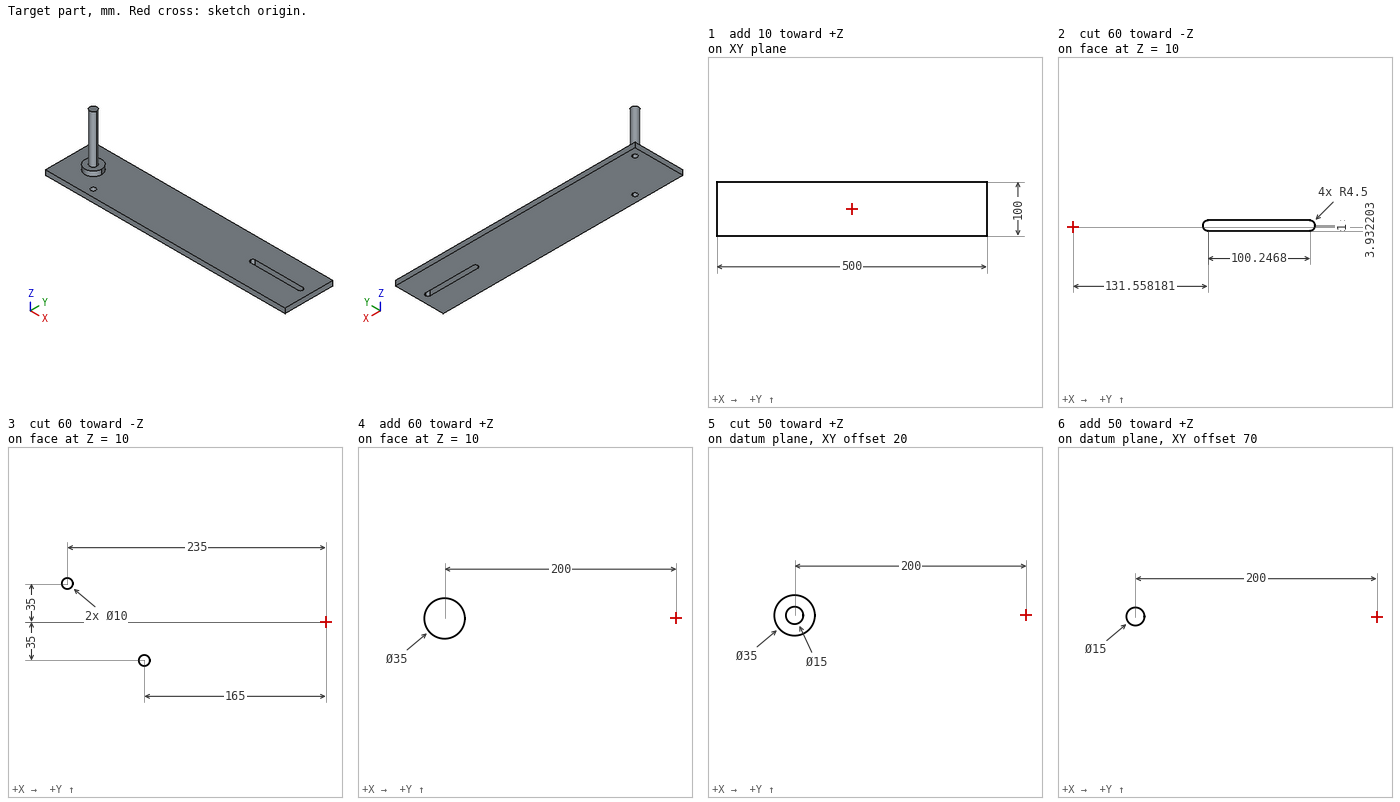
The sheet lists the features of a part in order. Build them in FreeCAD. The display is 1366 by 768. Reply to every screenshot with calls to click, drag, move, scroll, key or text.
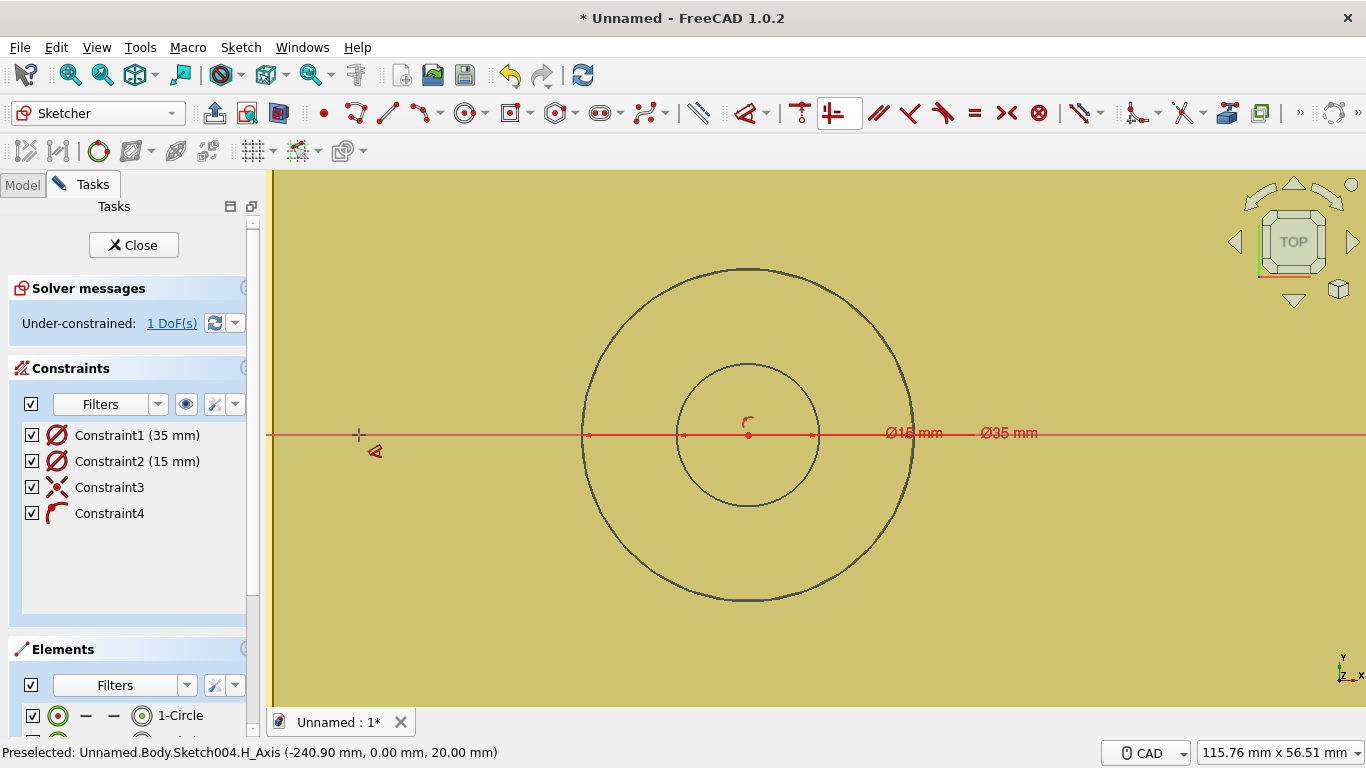
click(748, 435)
click(975, 469)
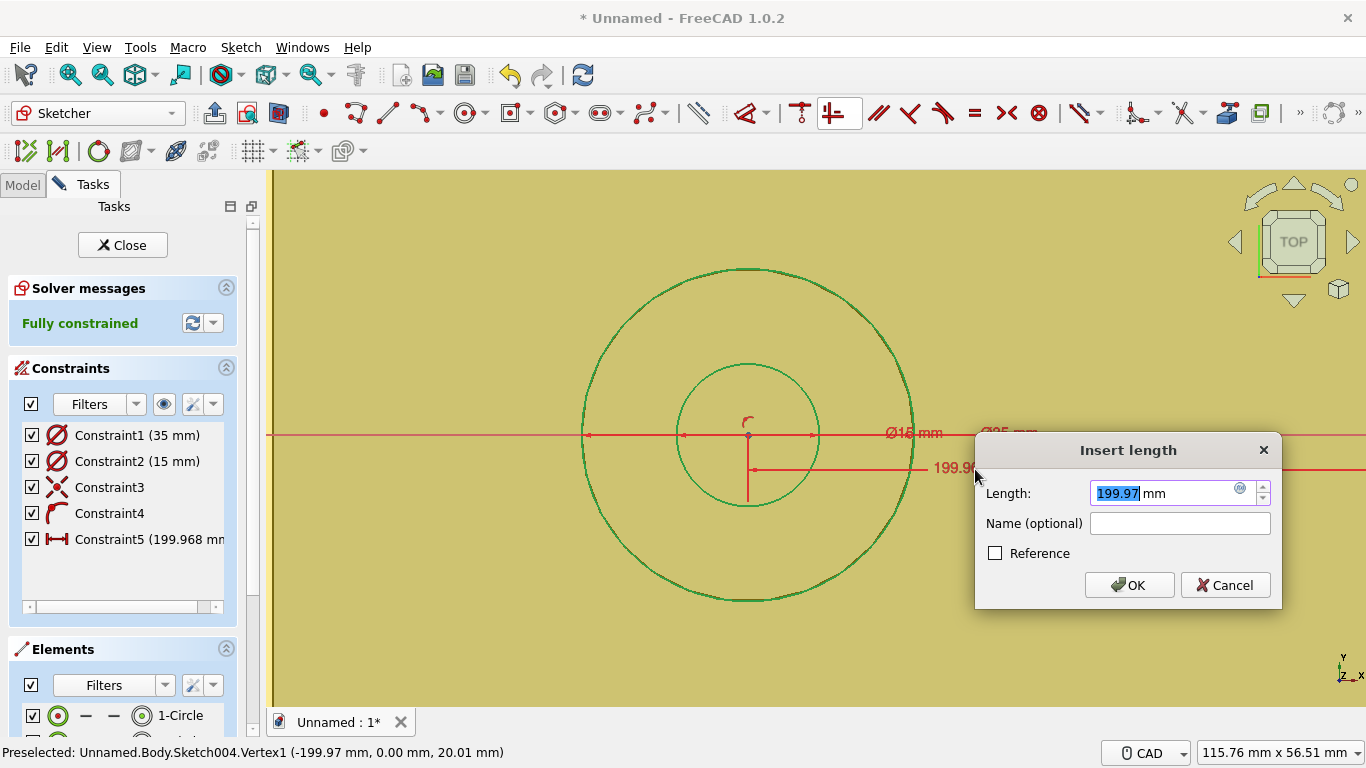
text(200)
key(Return)
key(Escape)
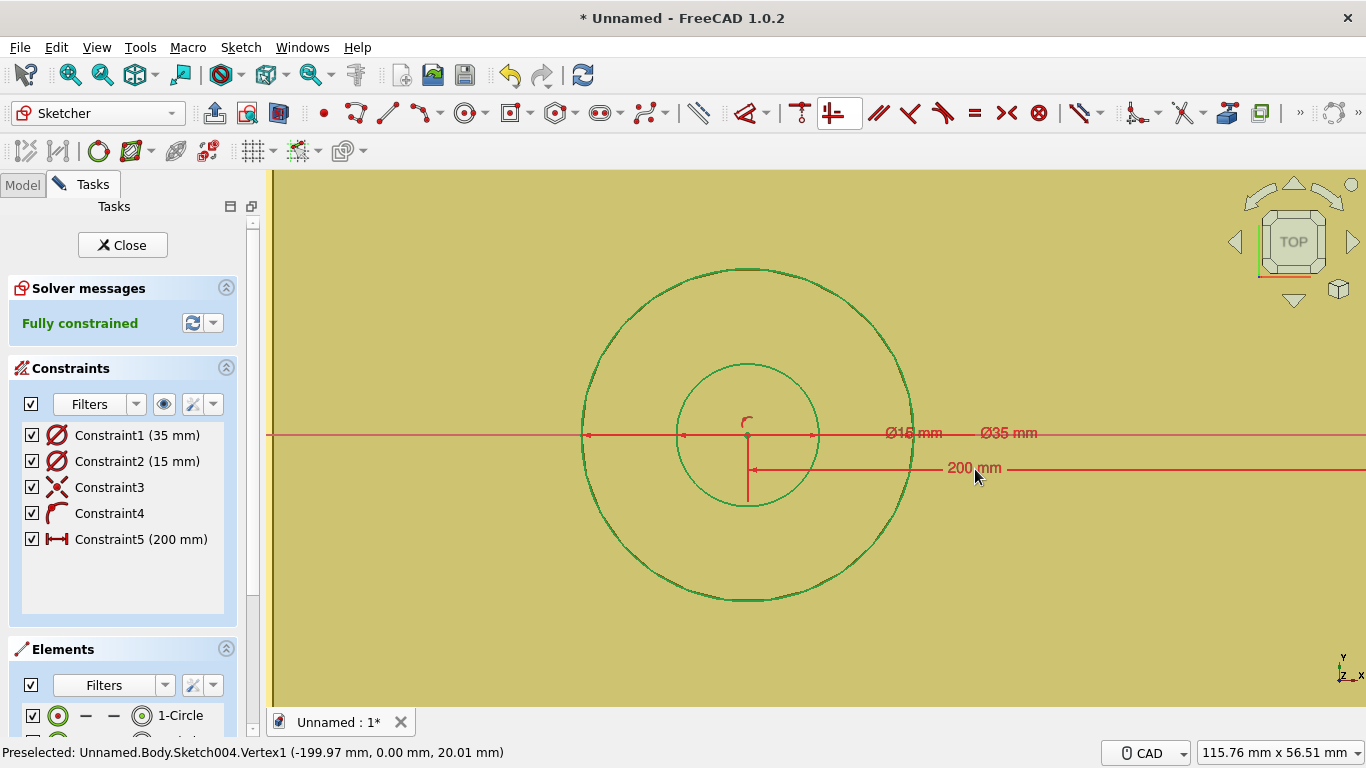
click(123, 245)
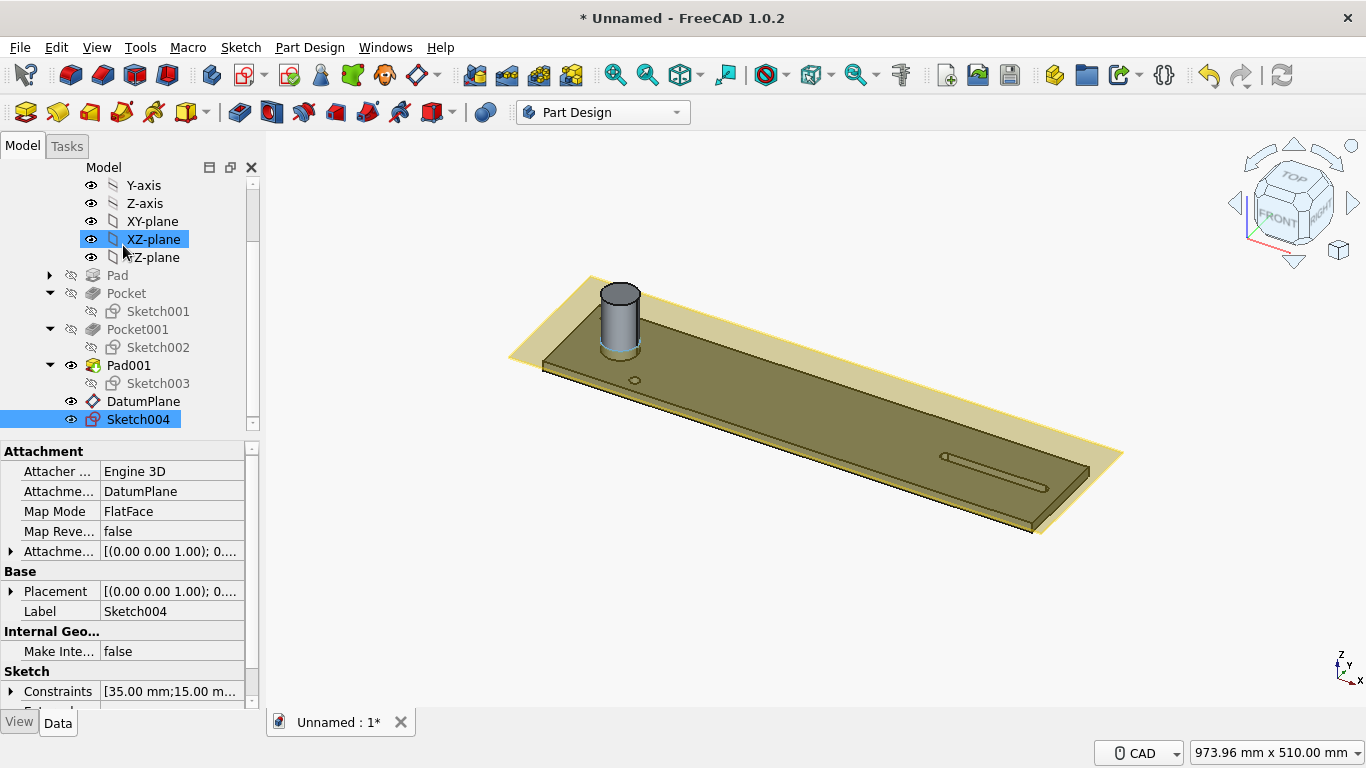
click(240, 112)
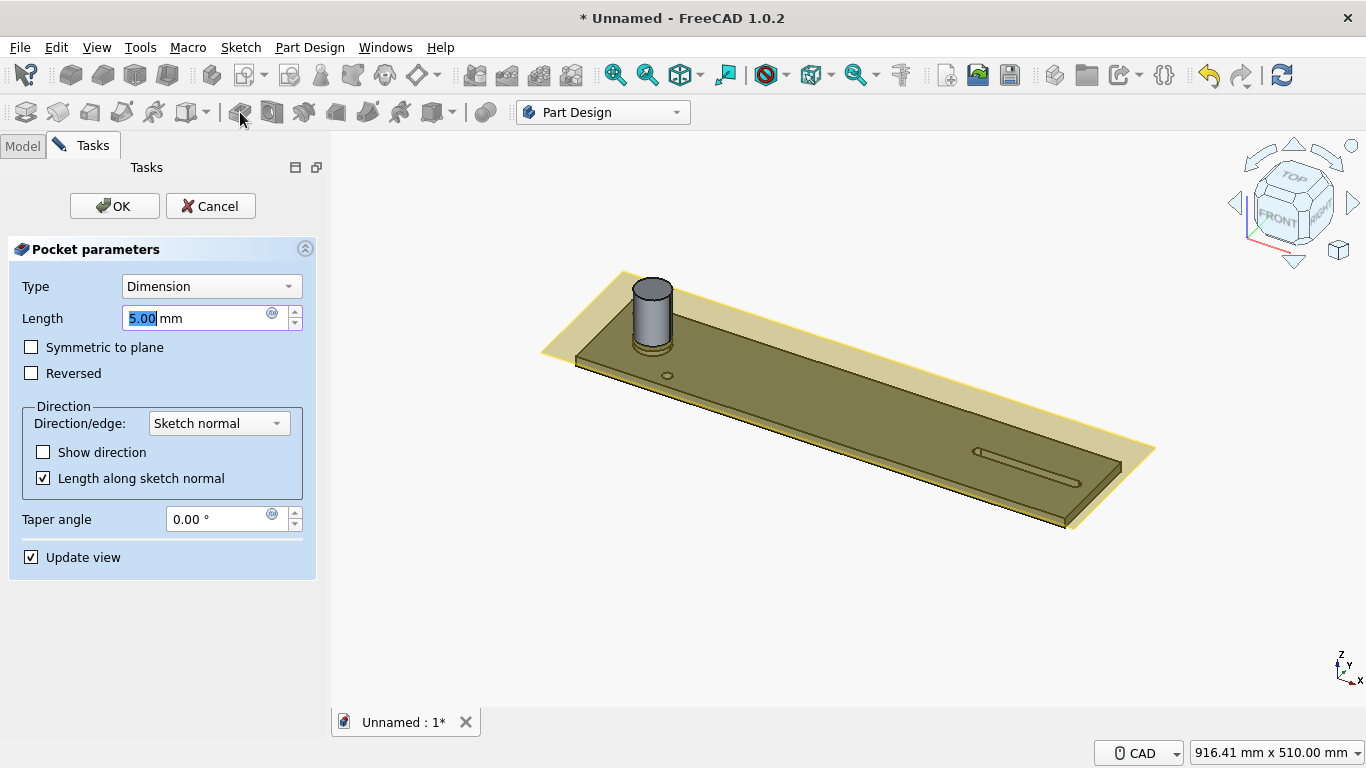
text(50)
key(Tab)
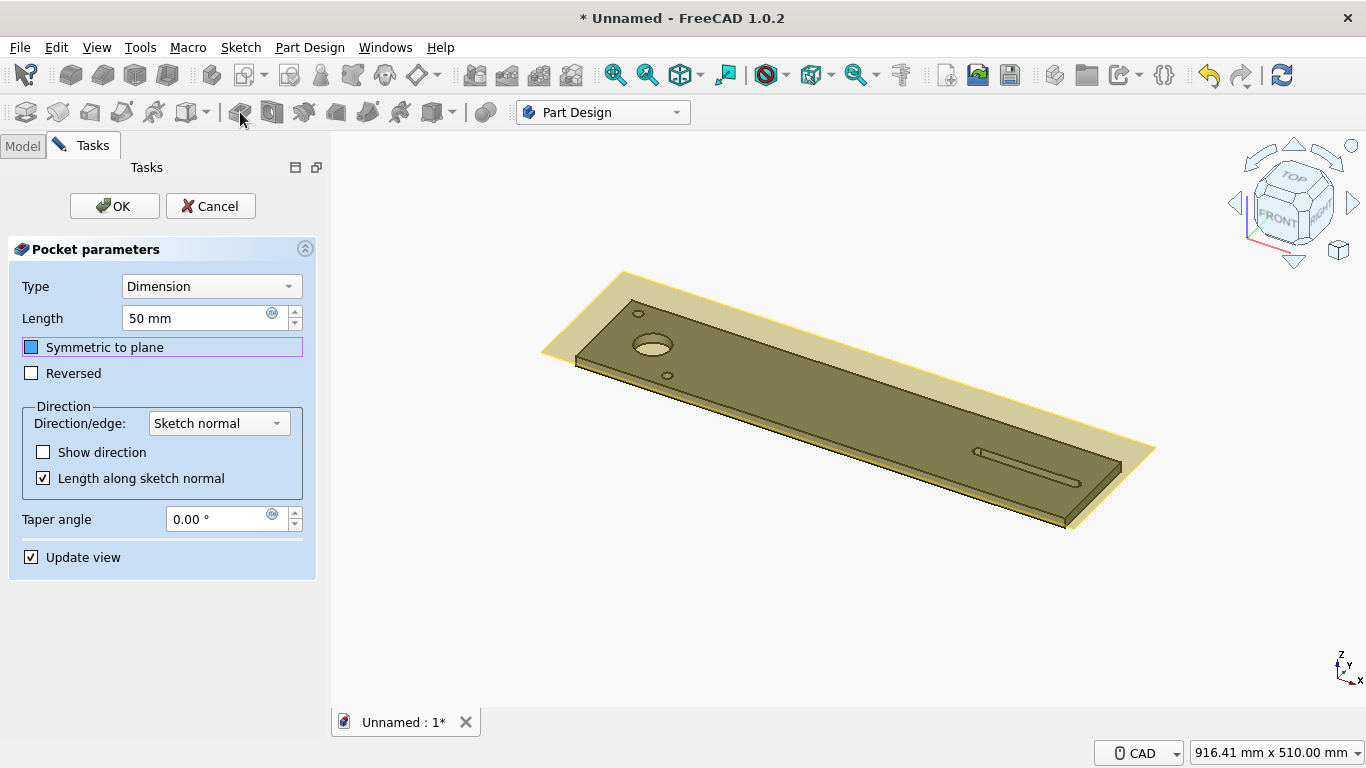
click(30, 373)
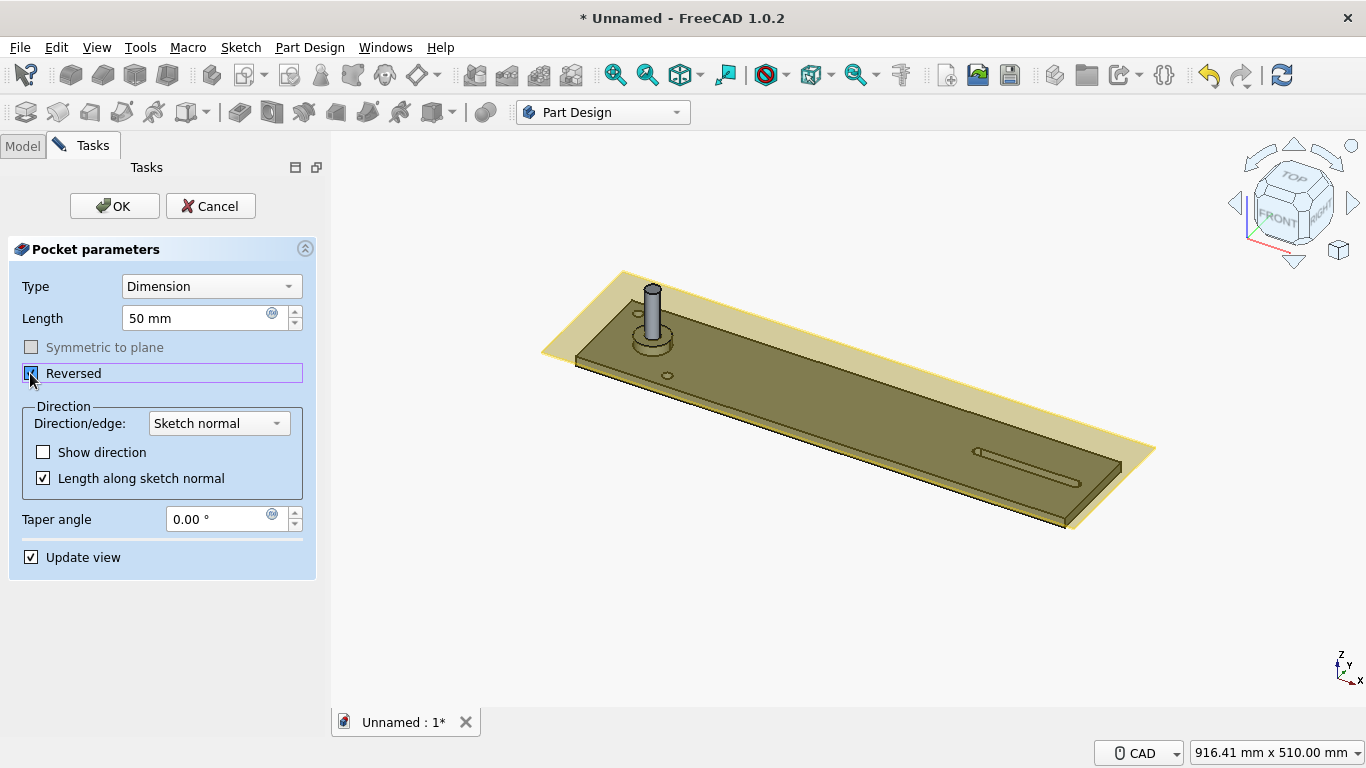
click(115, 206)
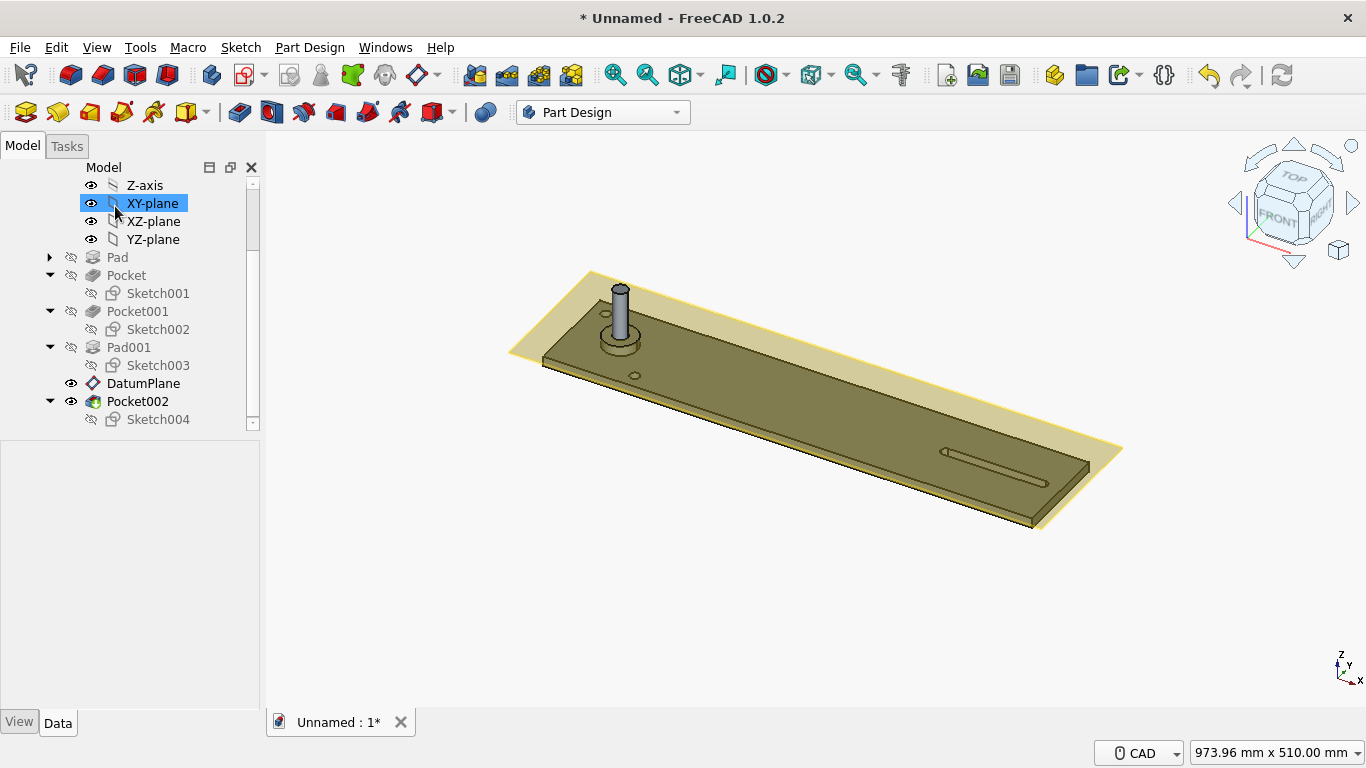
click(116, 383)
key(space)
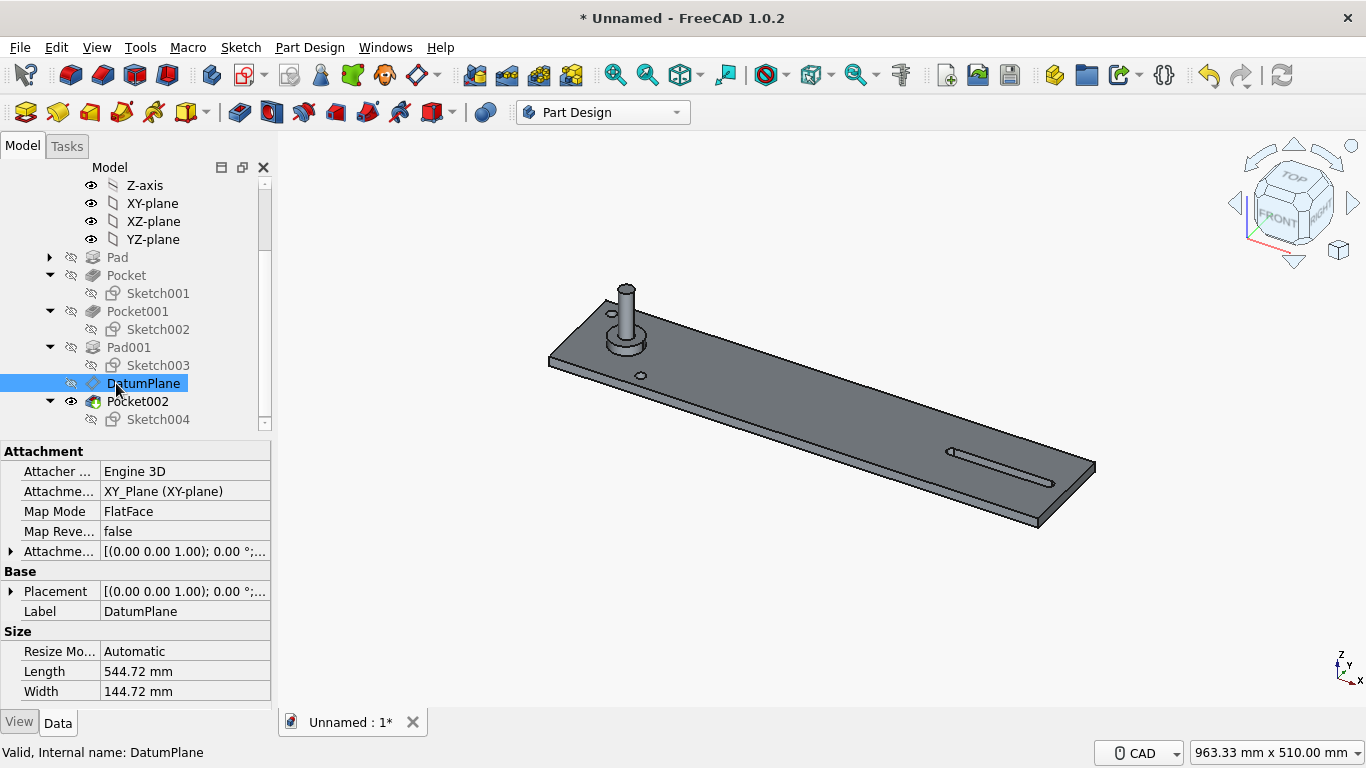
key(0)